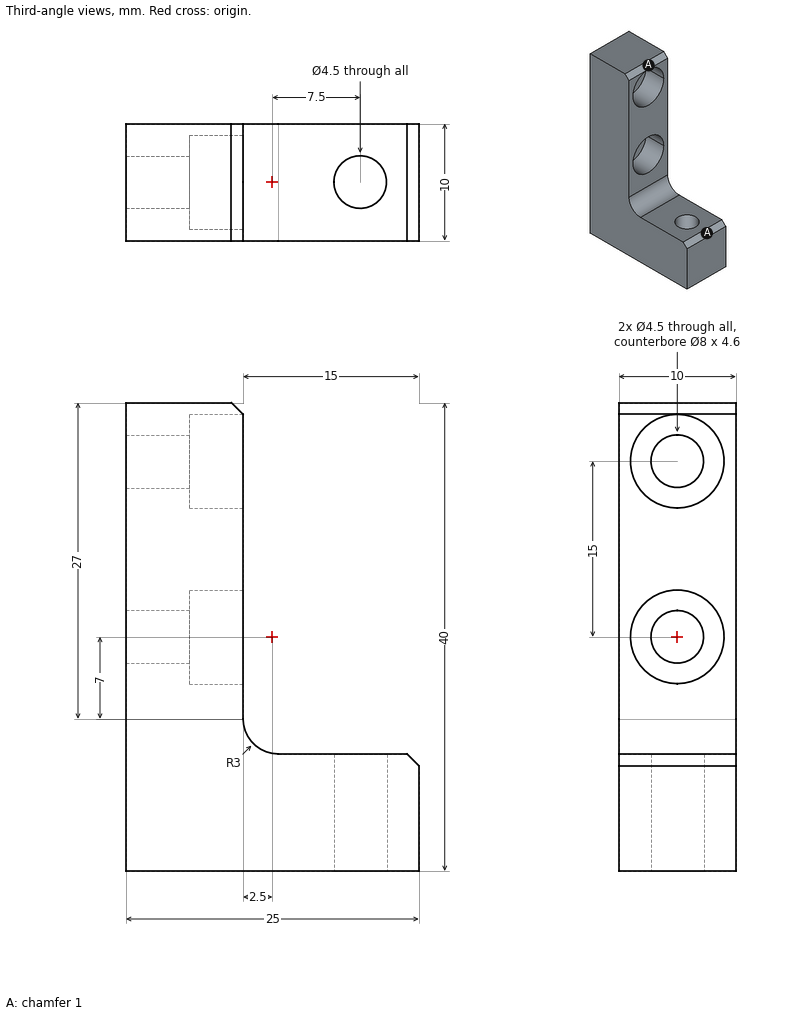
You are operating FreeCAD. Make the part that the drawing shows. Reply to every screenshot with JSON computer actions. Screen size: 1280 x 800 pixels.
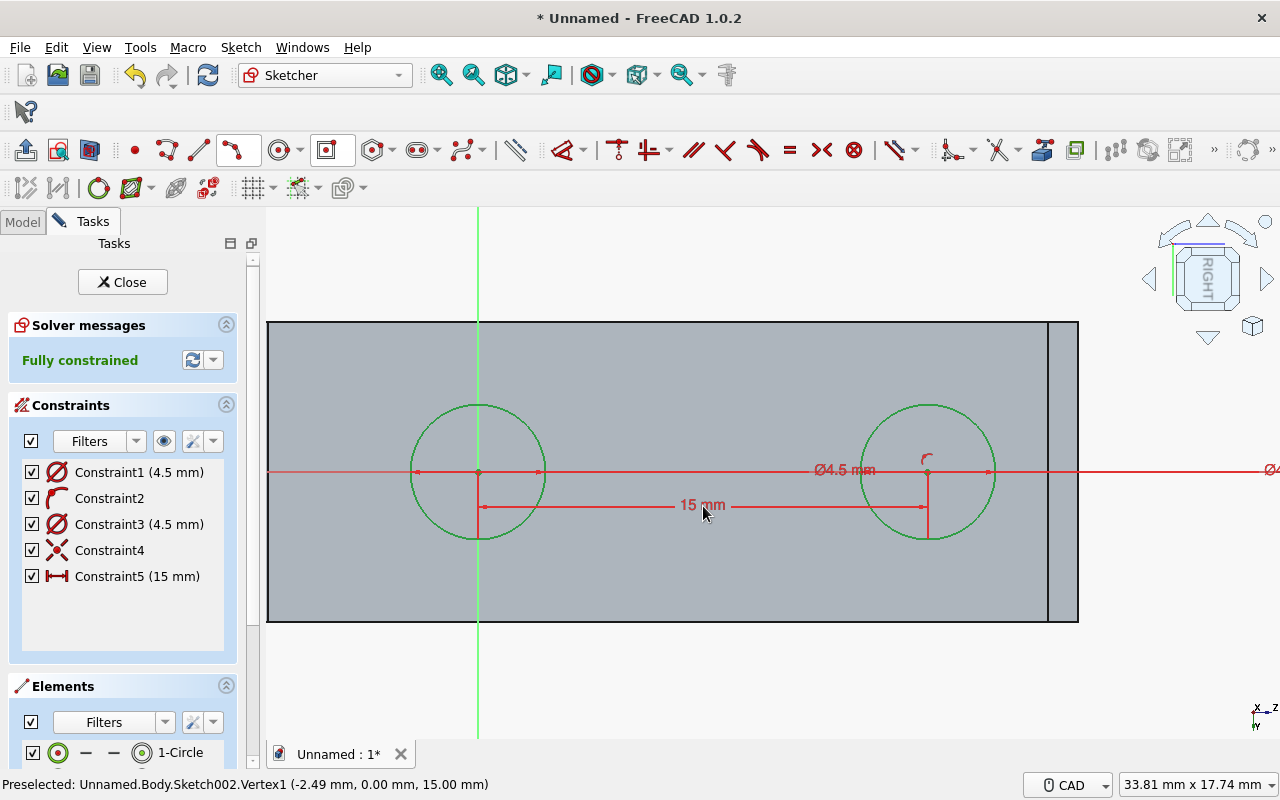
{"action": "left_click", "coordinate": [123, 282]}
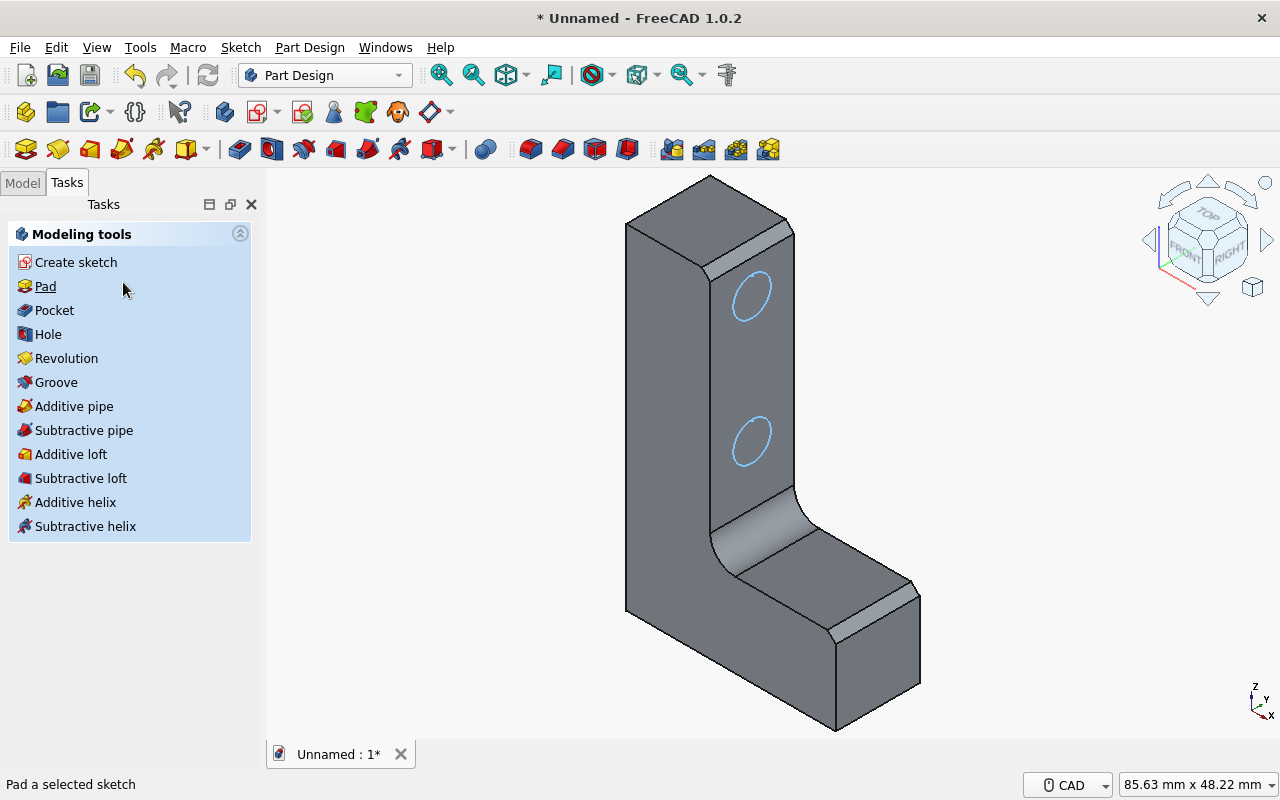
{"action": "left_click", "coordinate": [272, 150]}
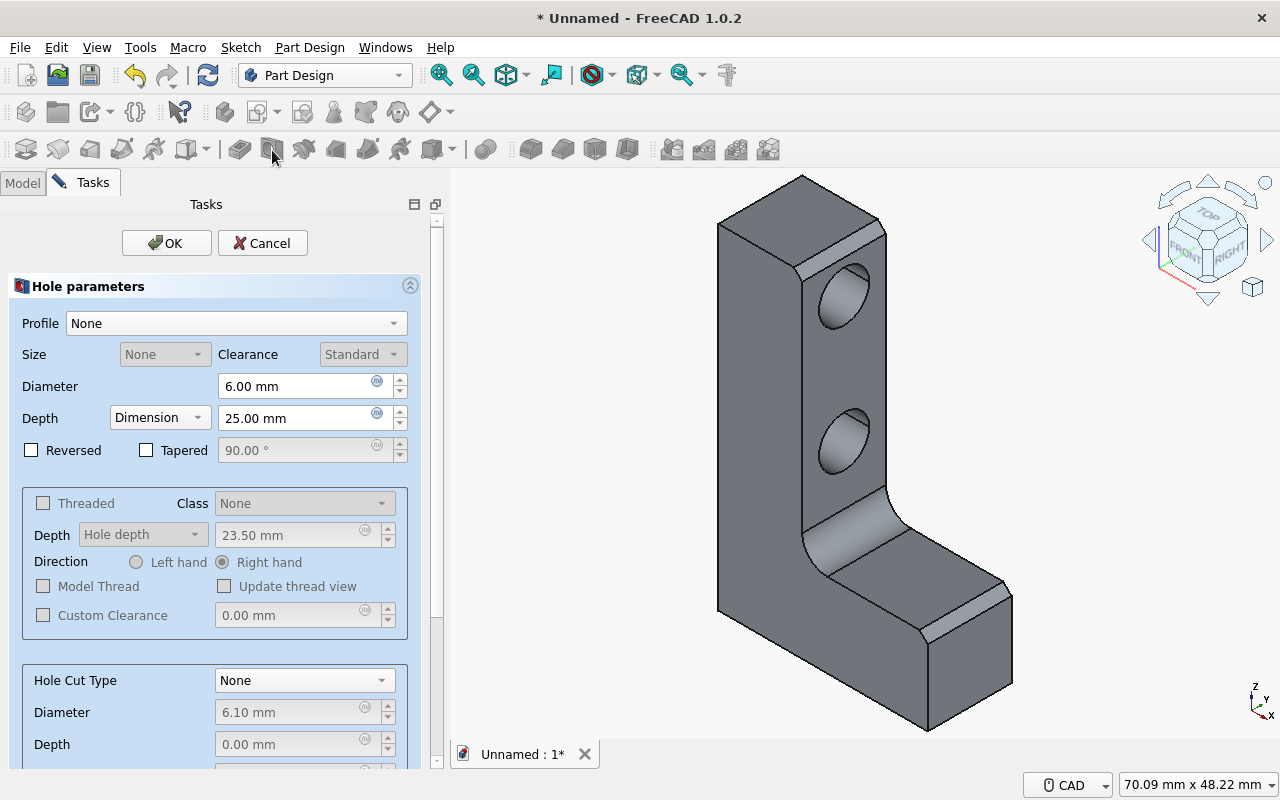
{"action": "triple_click", "coordinate": [305, 386]}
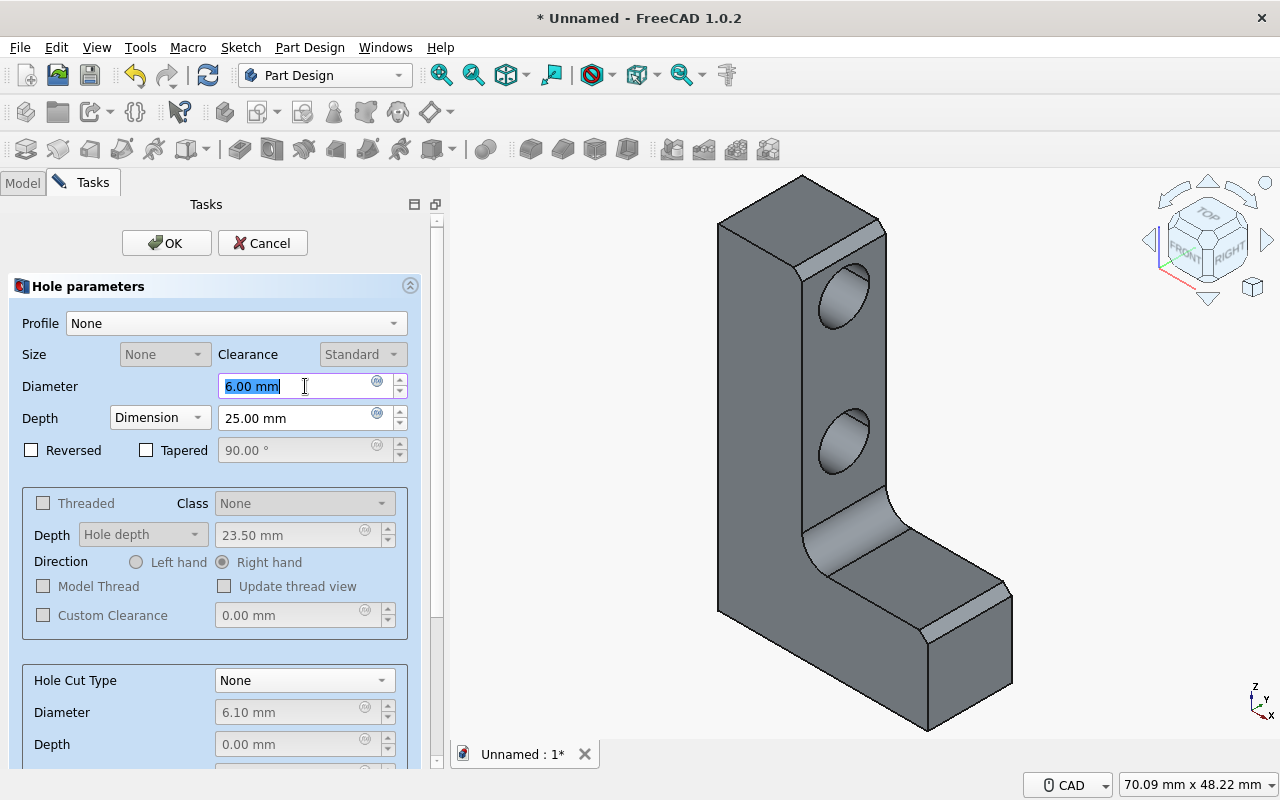
{"action": "type", "text": "4.5"}
{"action": "key", "text": "Tab"}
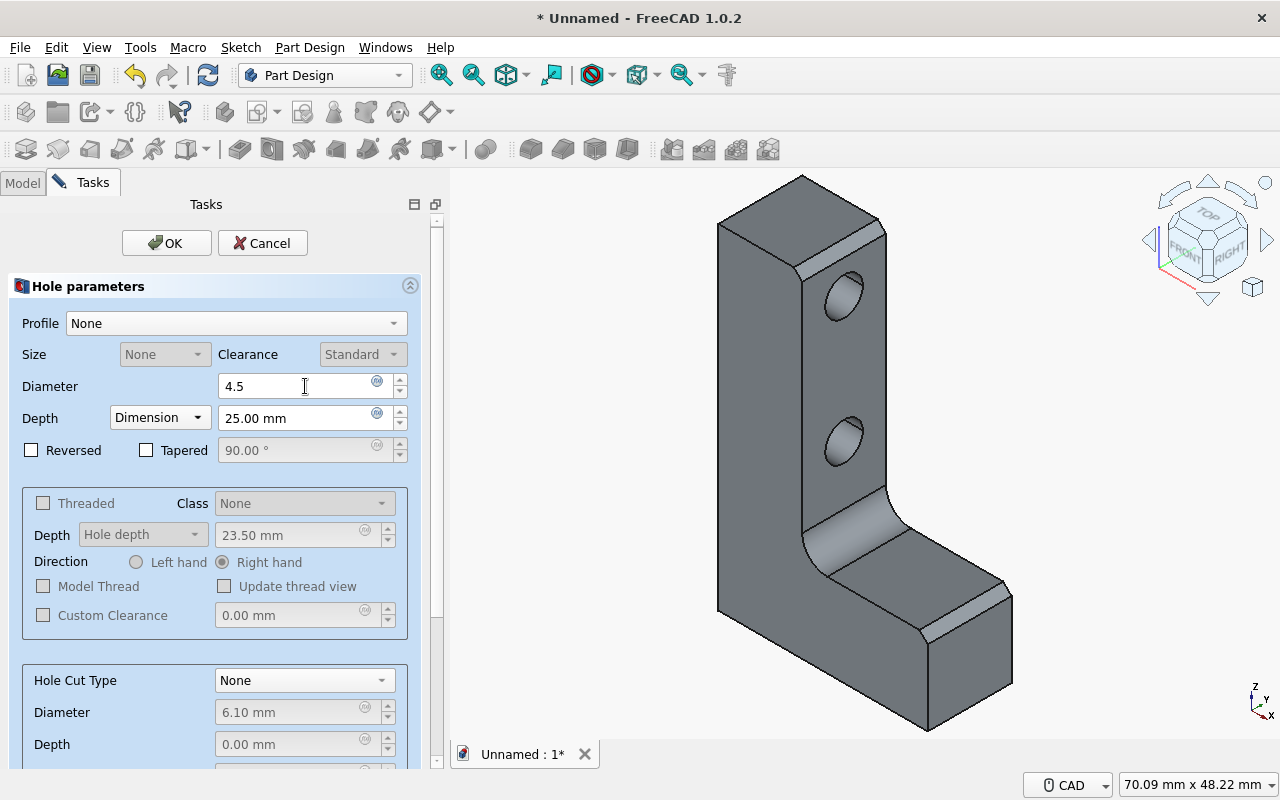
{"action": "left_click", "coordinate": [161, 418]}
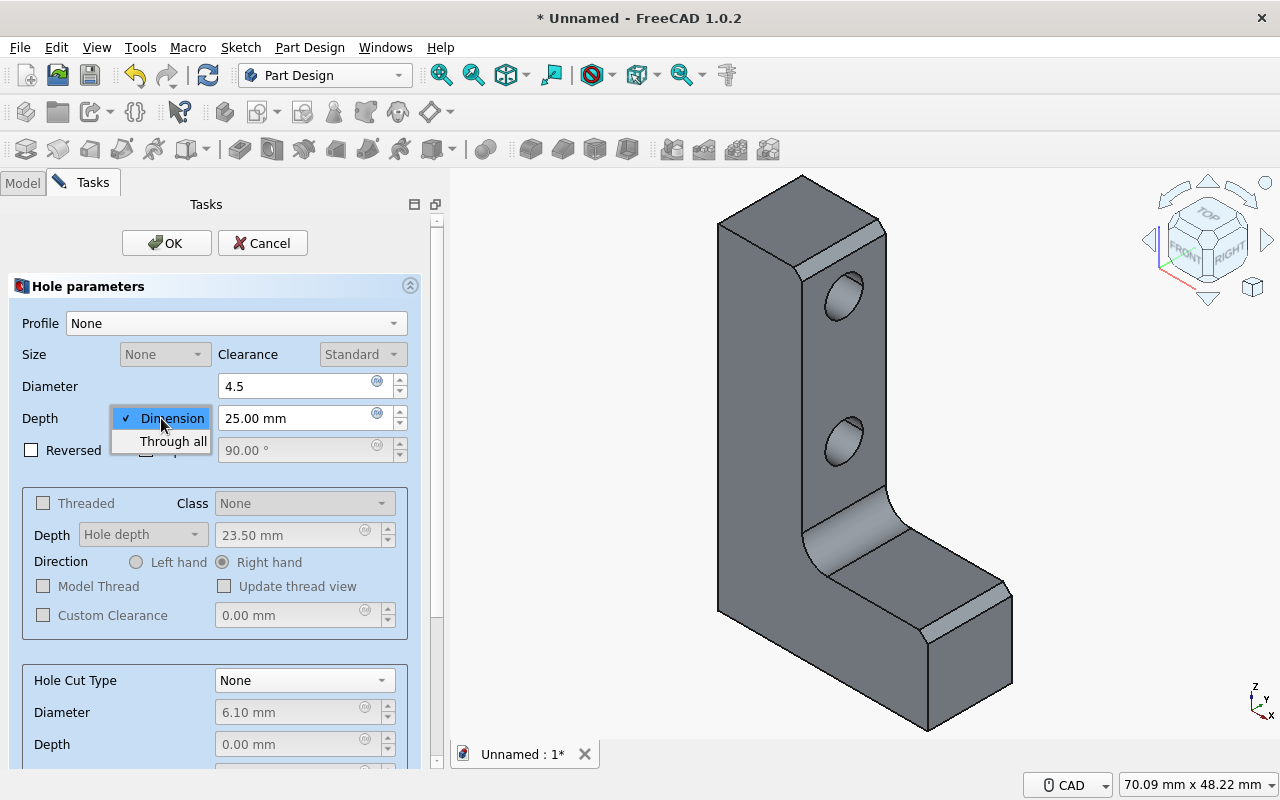
{"action": "left_click", "coordinate": [160, 442]}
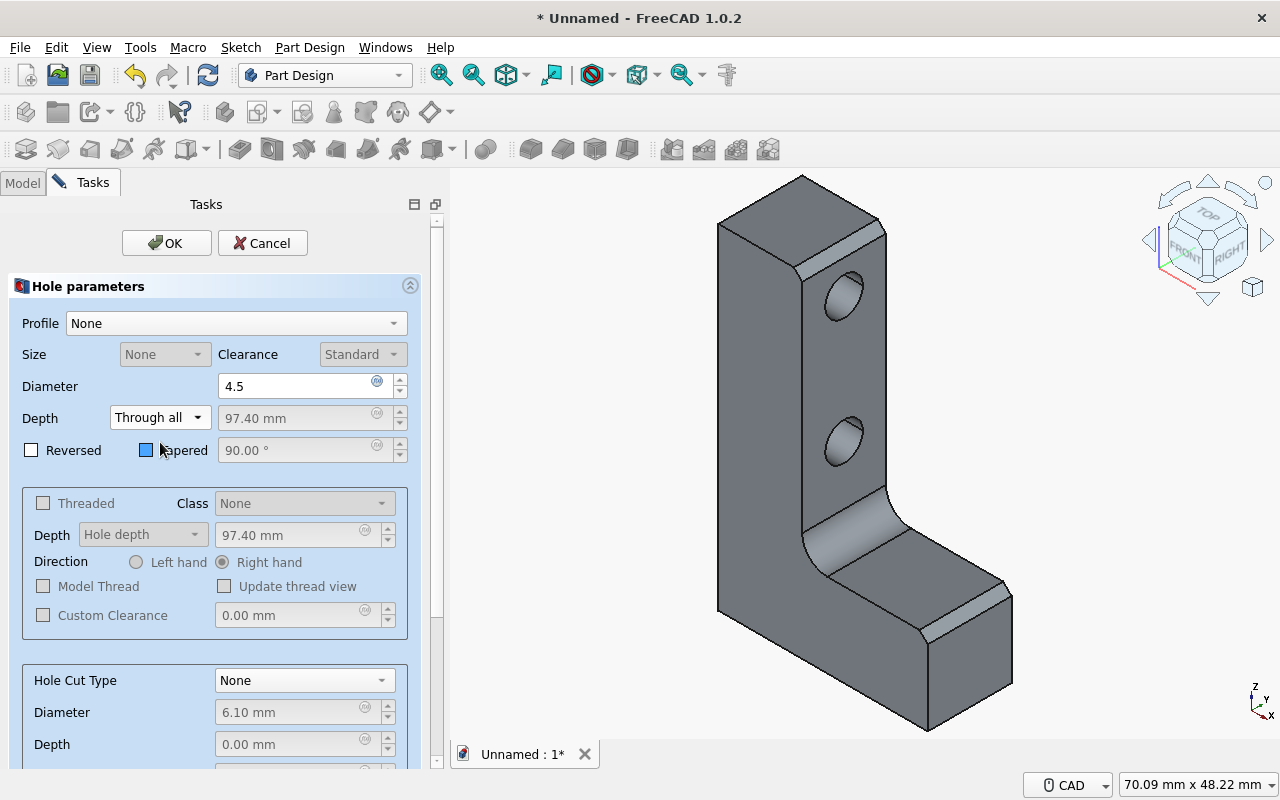
{"action": "left_click", "coordinate": [306, 680]}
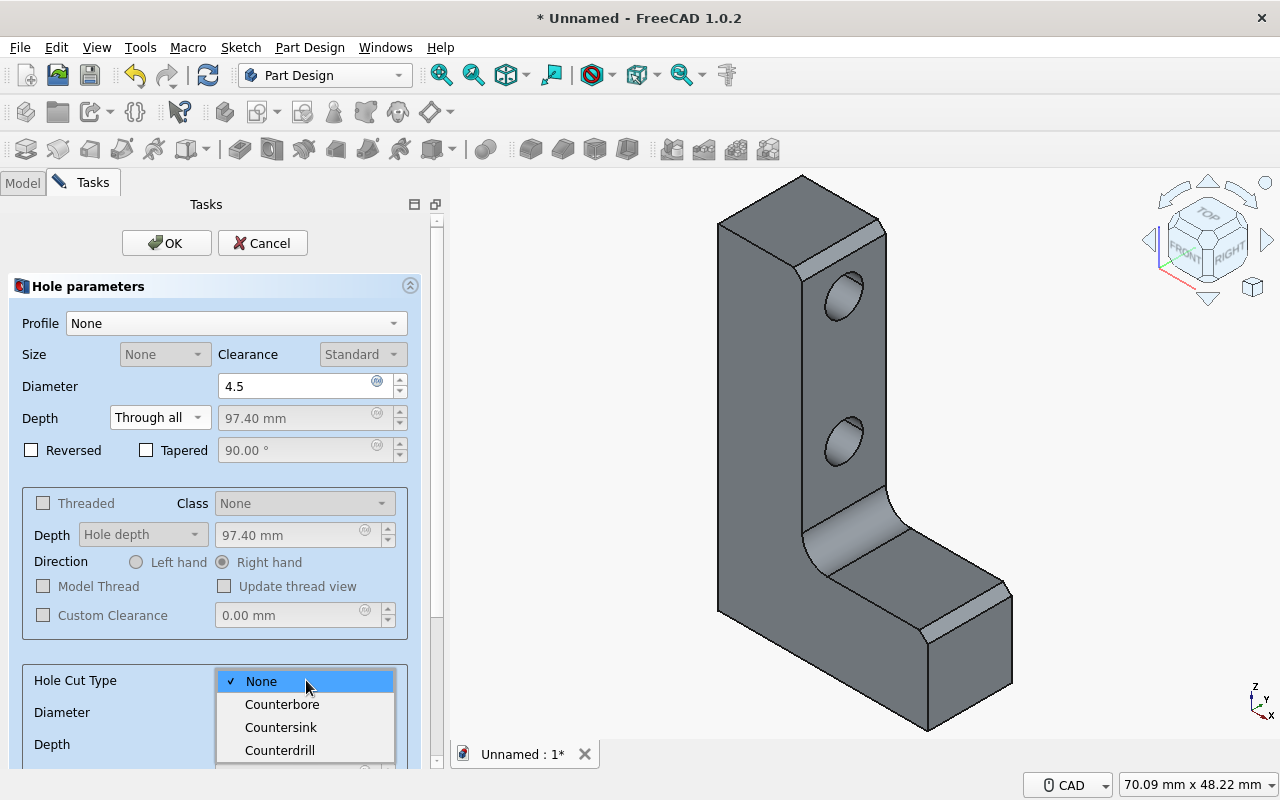
{"action": "left_click", "coordinate": [304, 704]}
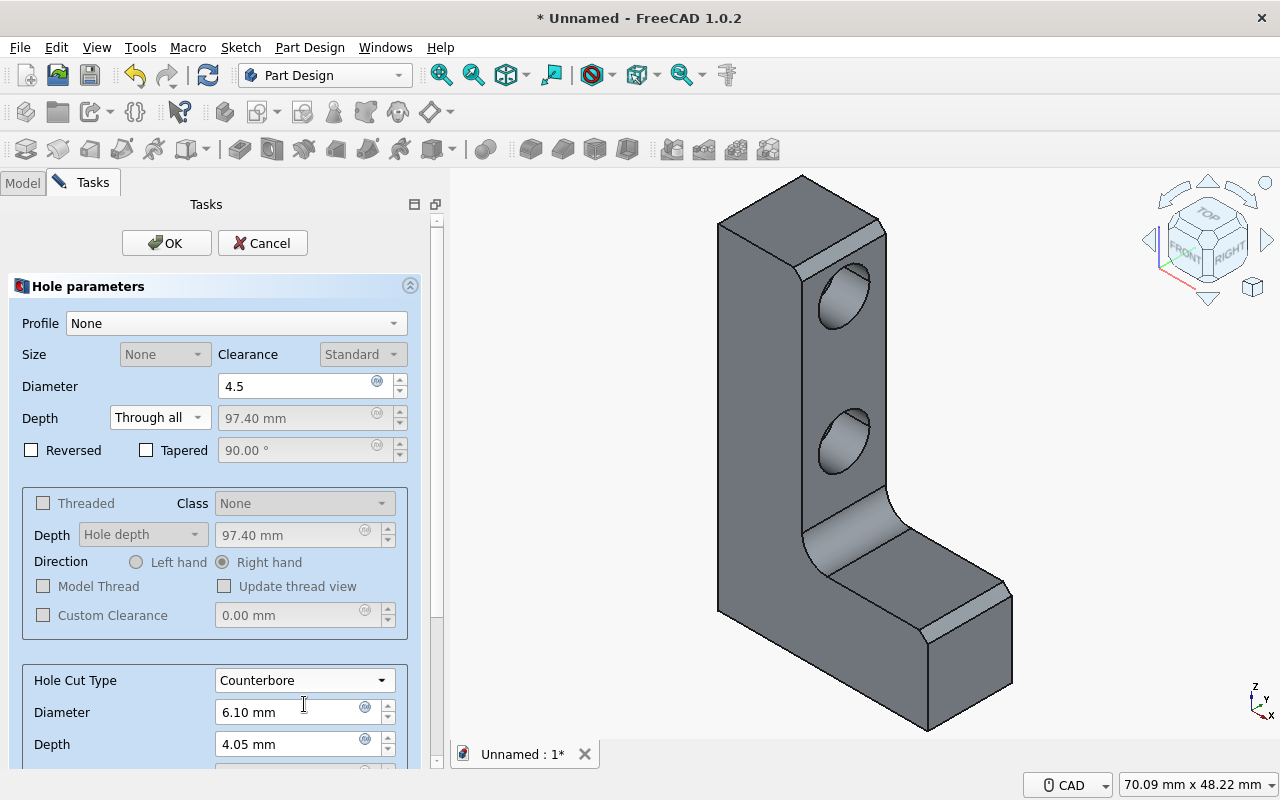
{"action": "triple_click", "coordinate": [298, 712]}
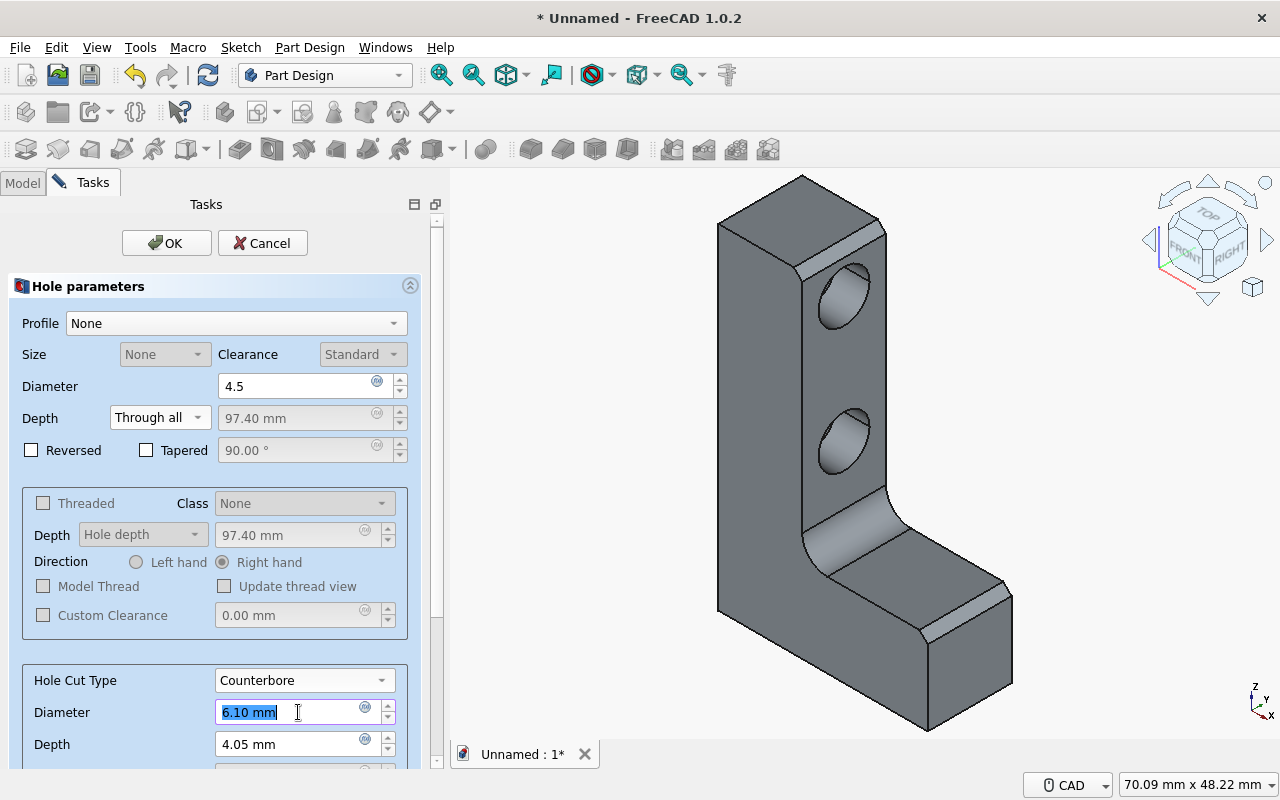
{"action": "type", "text": "8"}
{"action": "key", "text": "Tab"}